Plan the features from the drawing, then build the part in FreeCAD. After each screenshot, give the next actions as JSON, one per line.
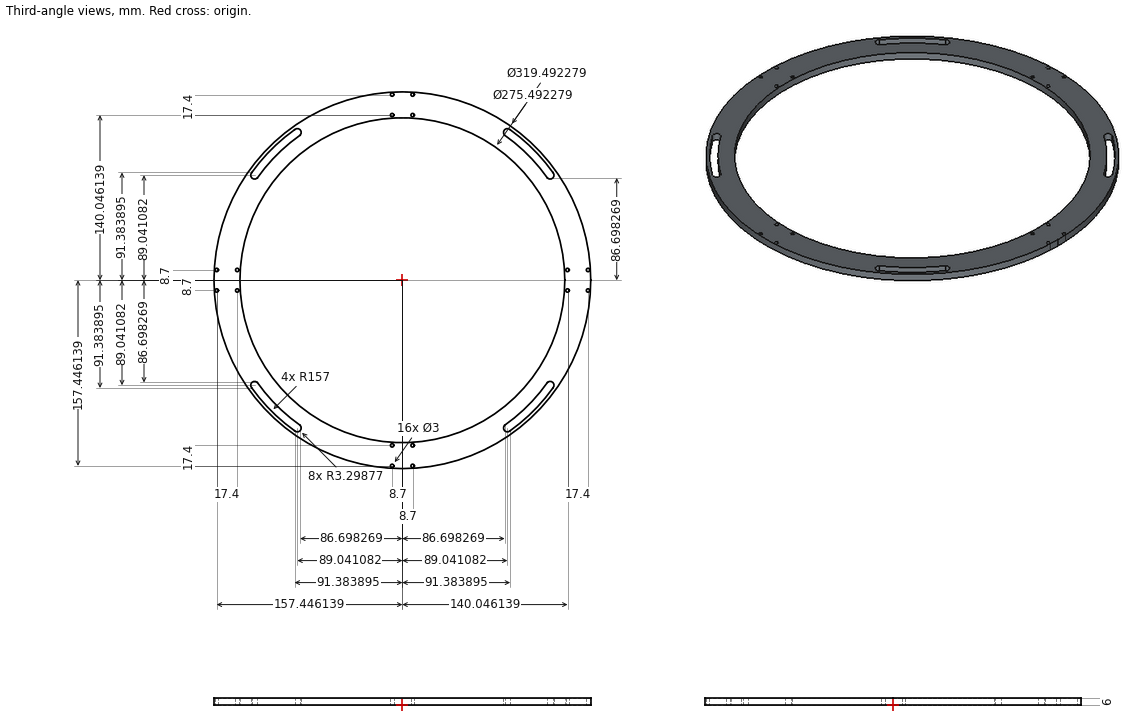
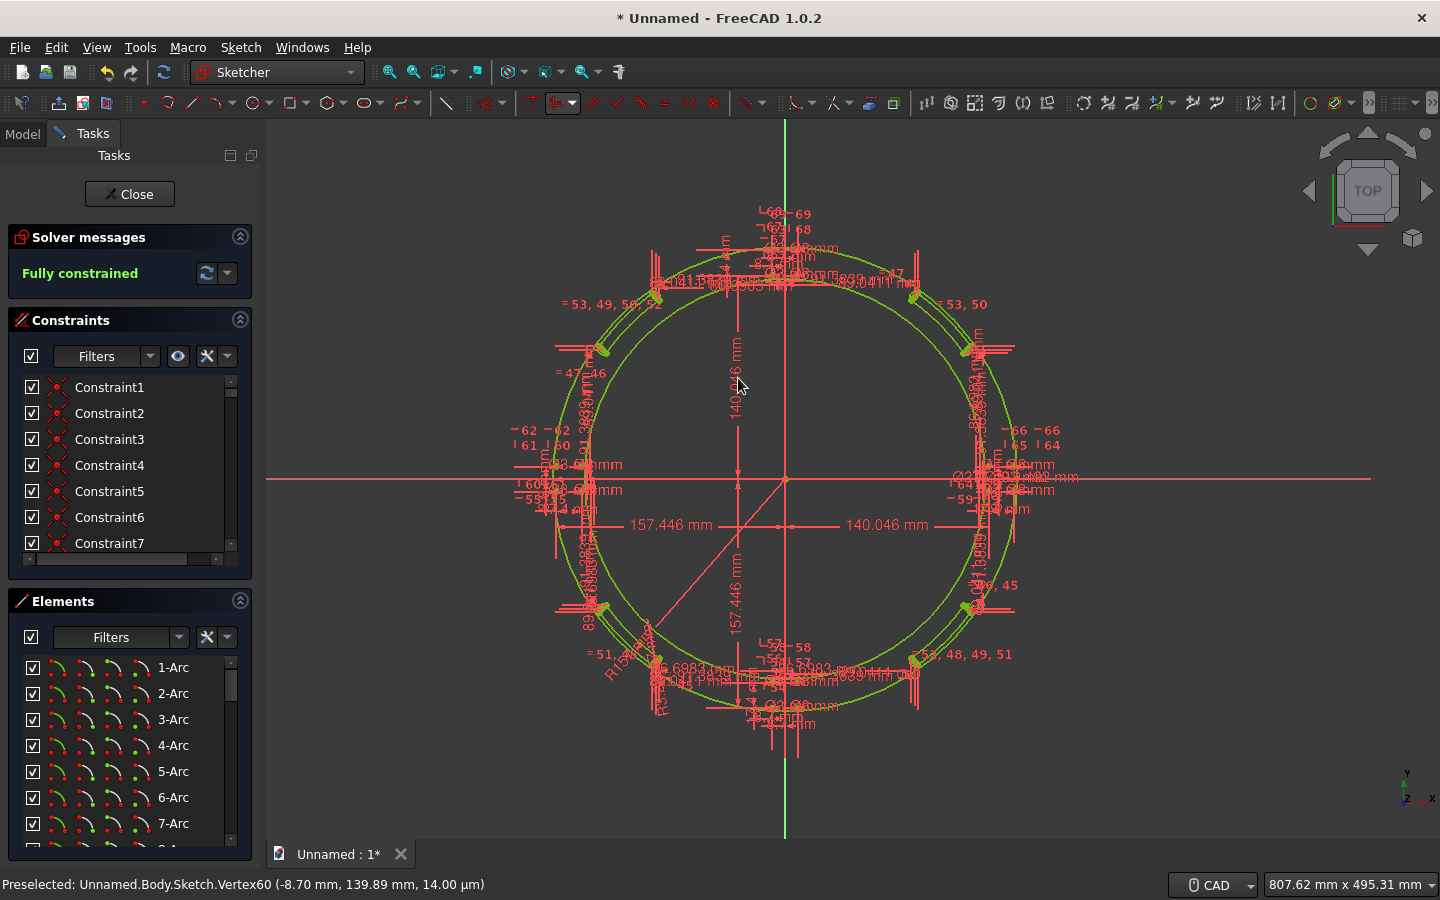
{"action": "left_click", "coordinate": [130, 194]}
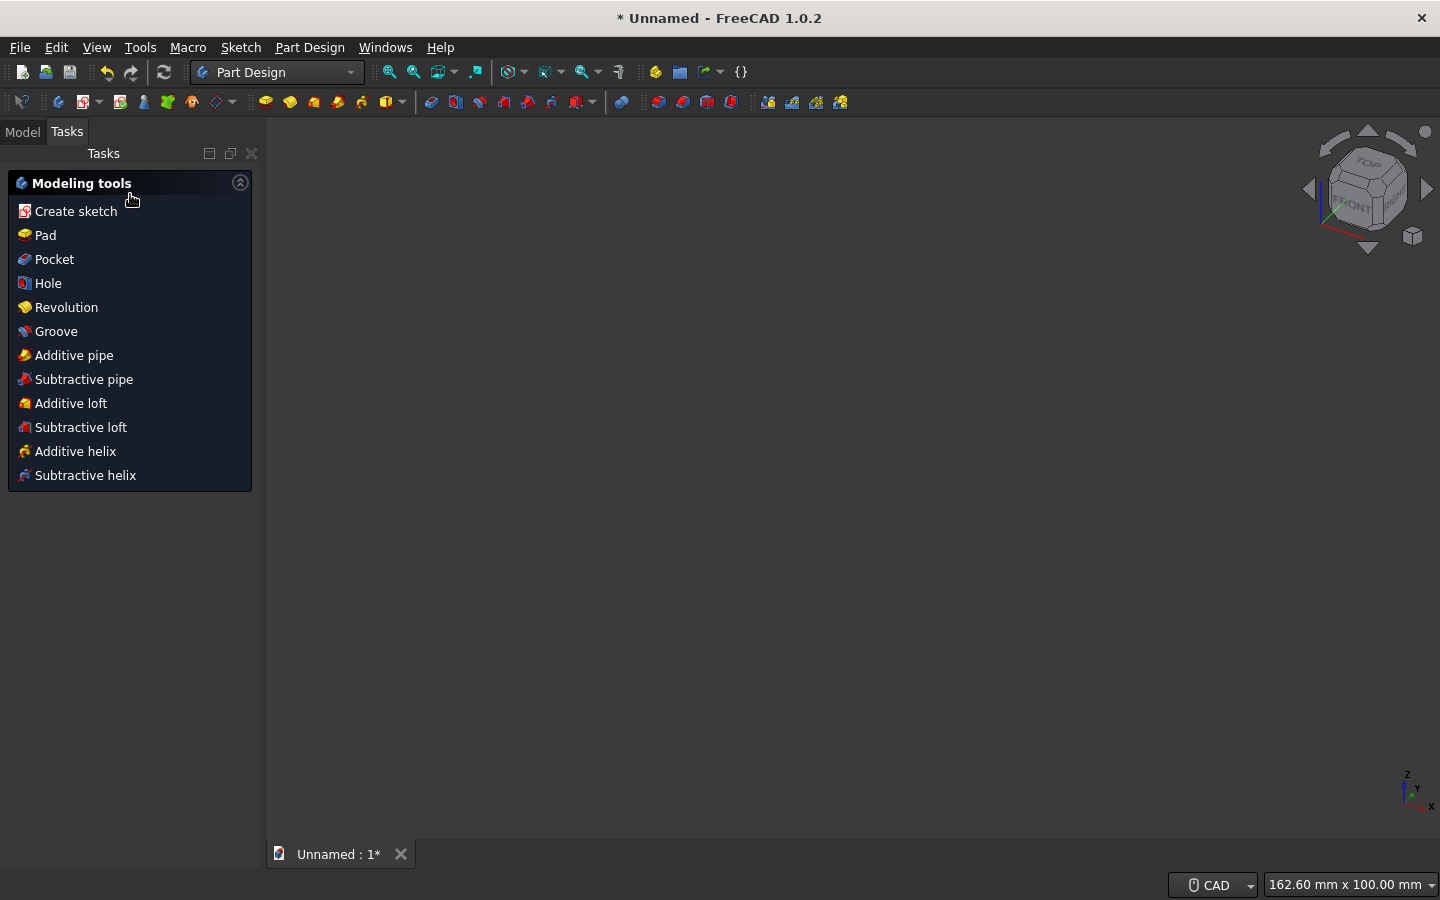
{"action": "left_click", "coordinate": [266, 102]}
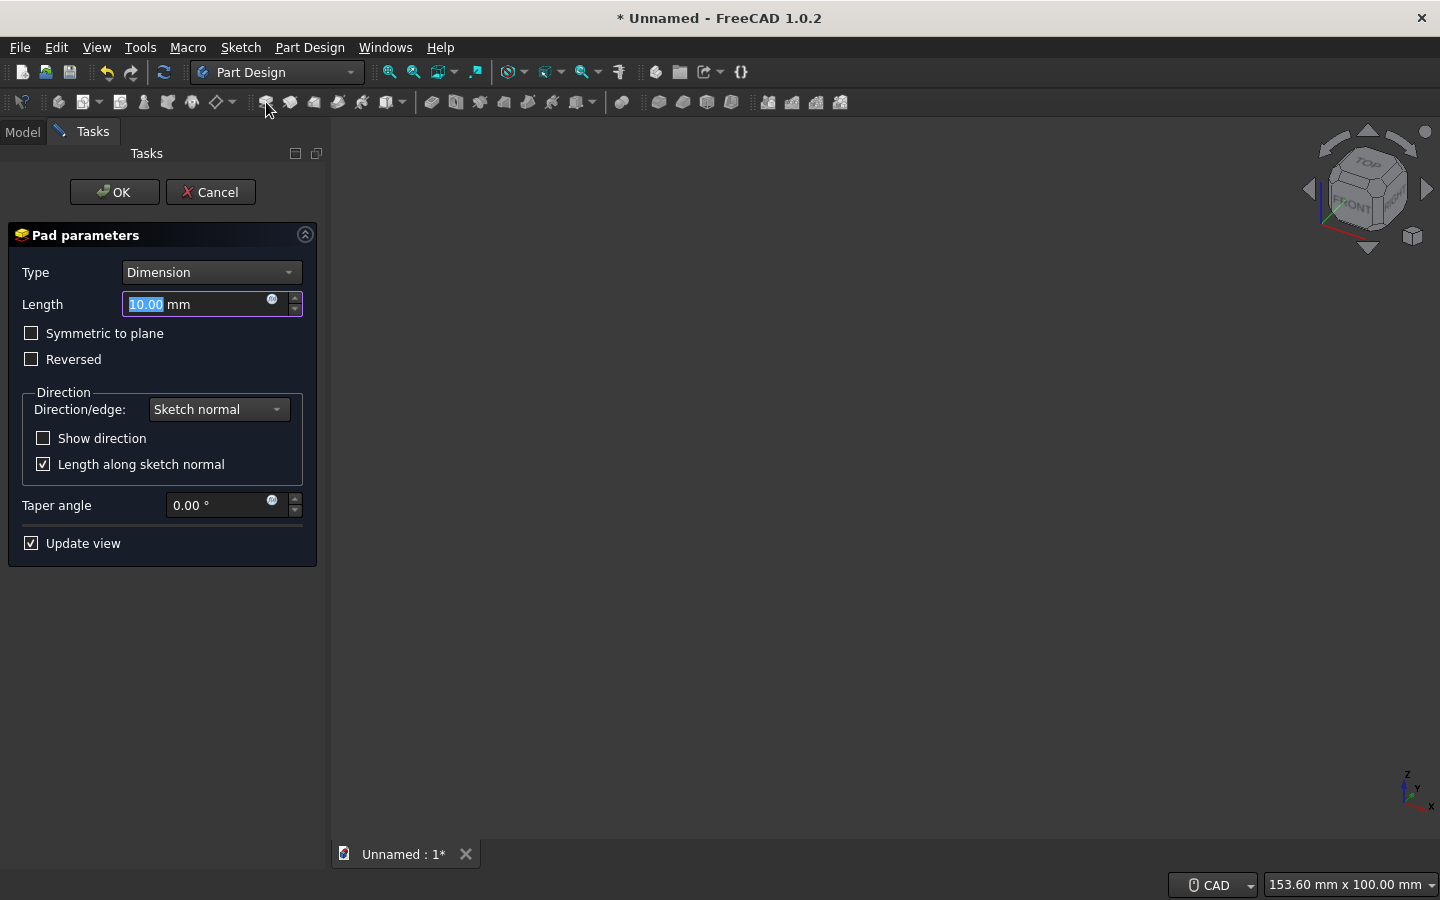
{"action": "type", "text": "6"}
{"action": "key", "text": "Tab"}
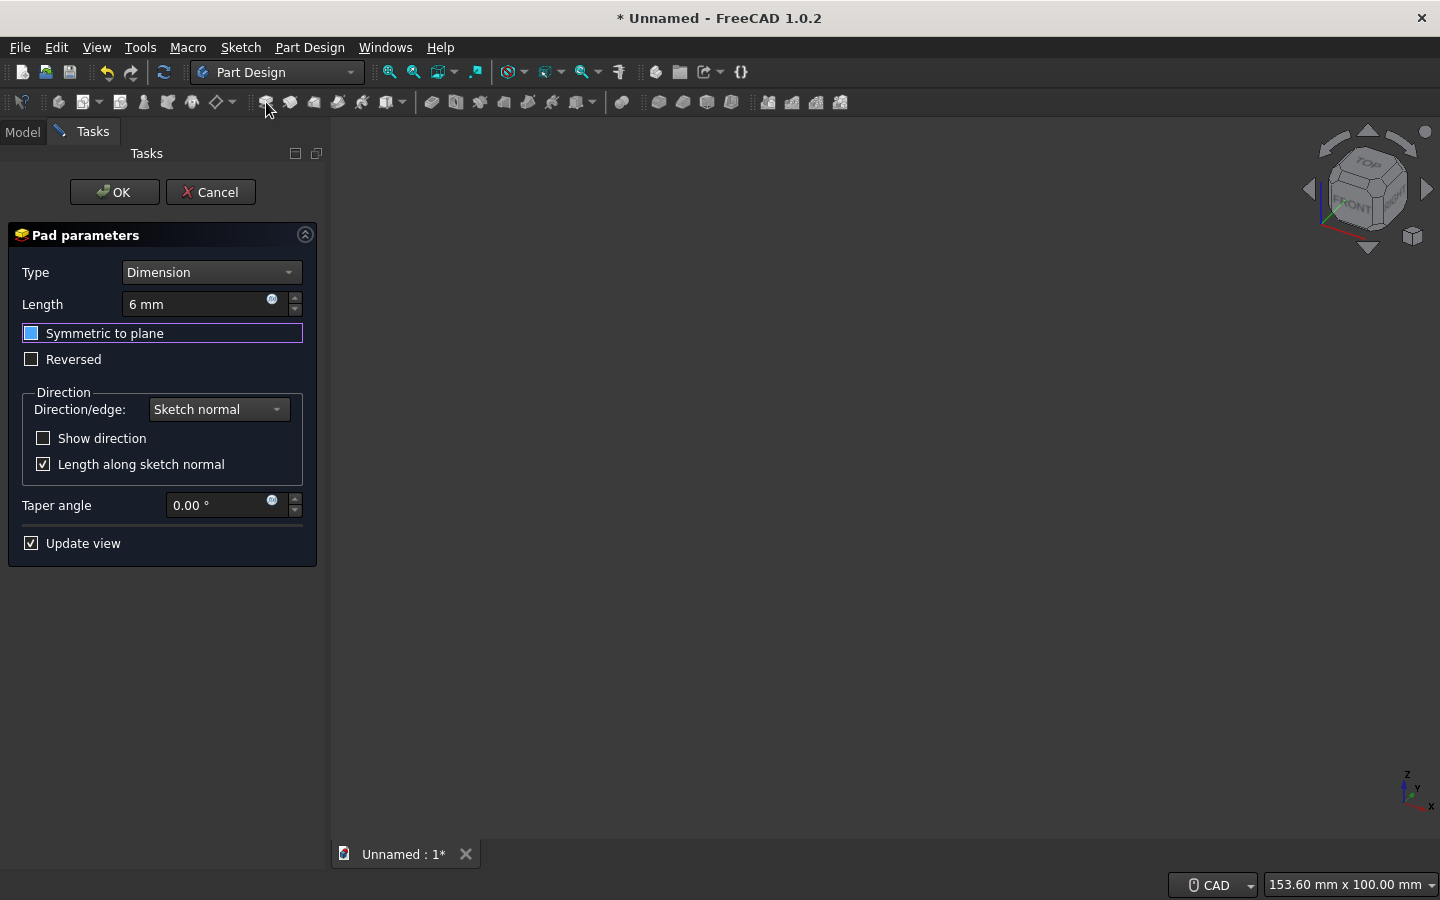
{"action": "left_click", "coordinate": [115, 192]}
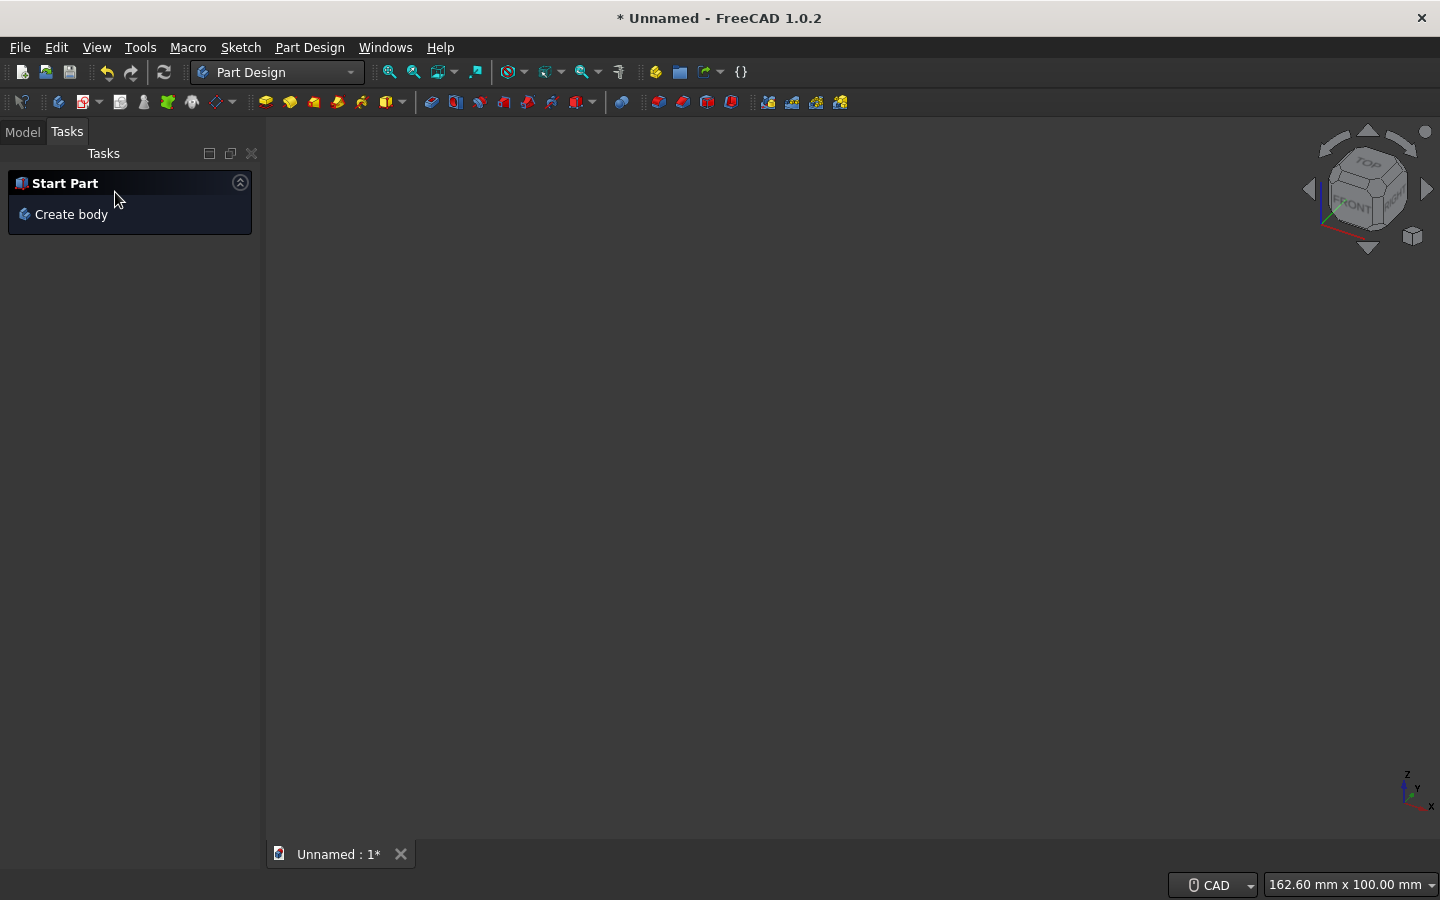
{"action": "key", "text": "0"}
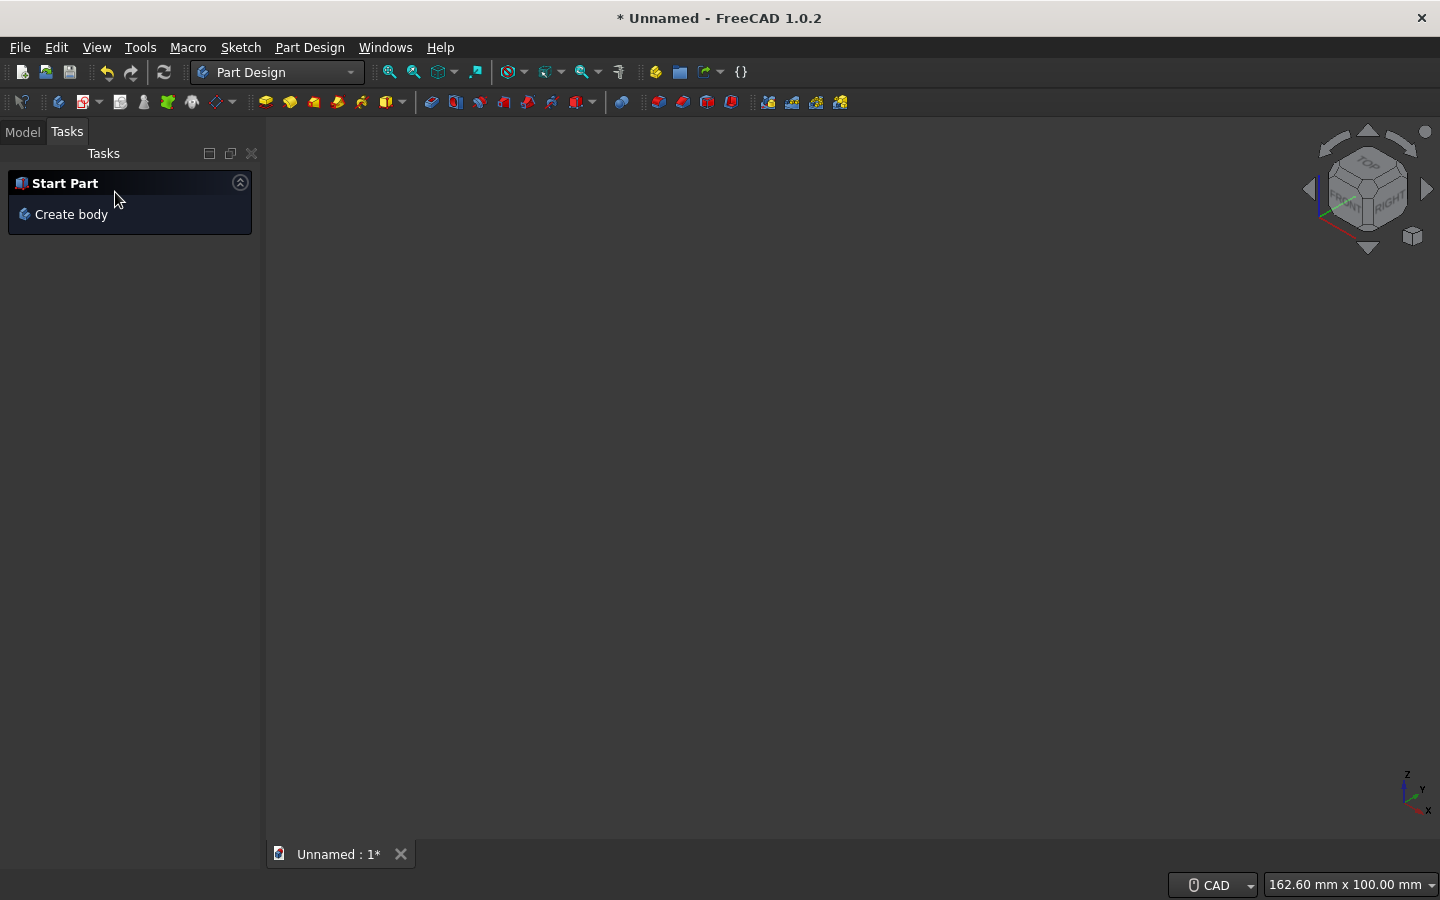
{"action": "key", "text": "v f"}